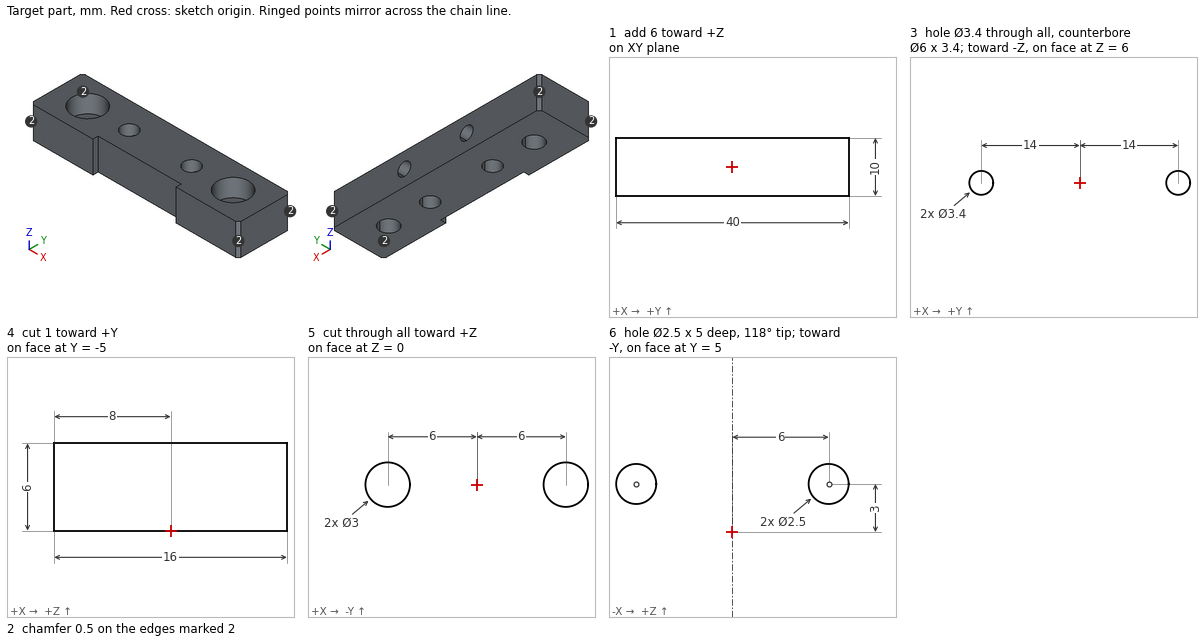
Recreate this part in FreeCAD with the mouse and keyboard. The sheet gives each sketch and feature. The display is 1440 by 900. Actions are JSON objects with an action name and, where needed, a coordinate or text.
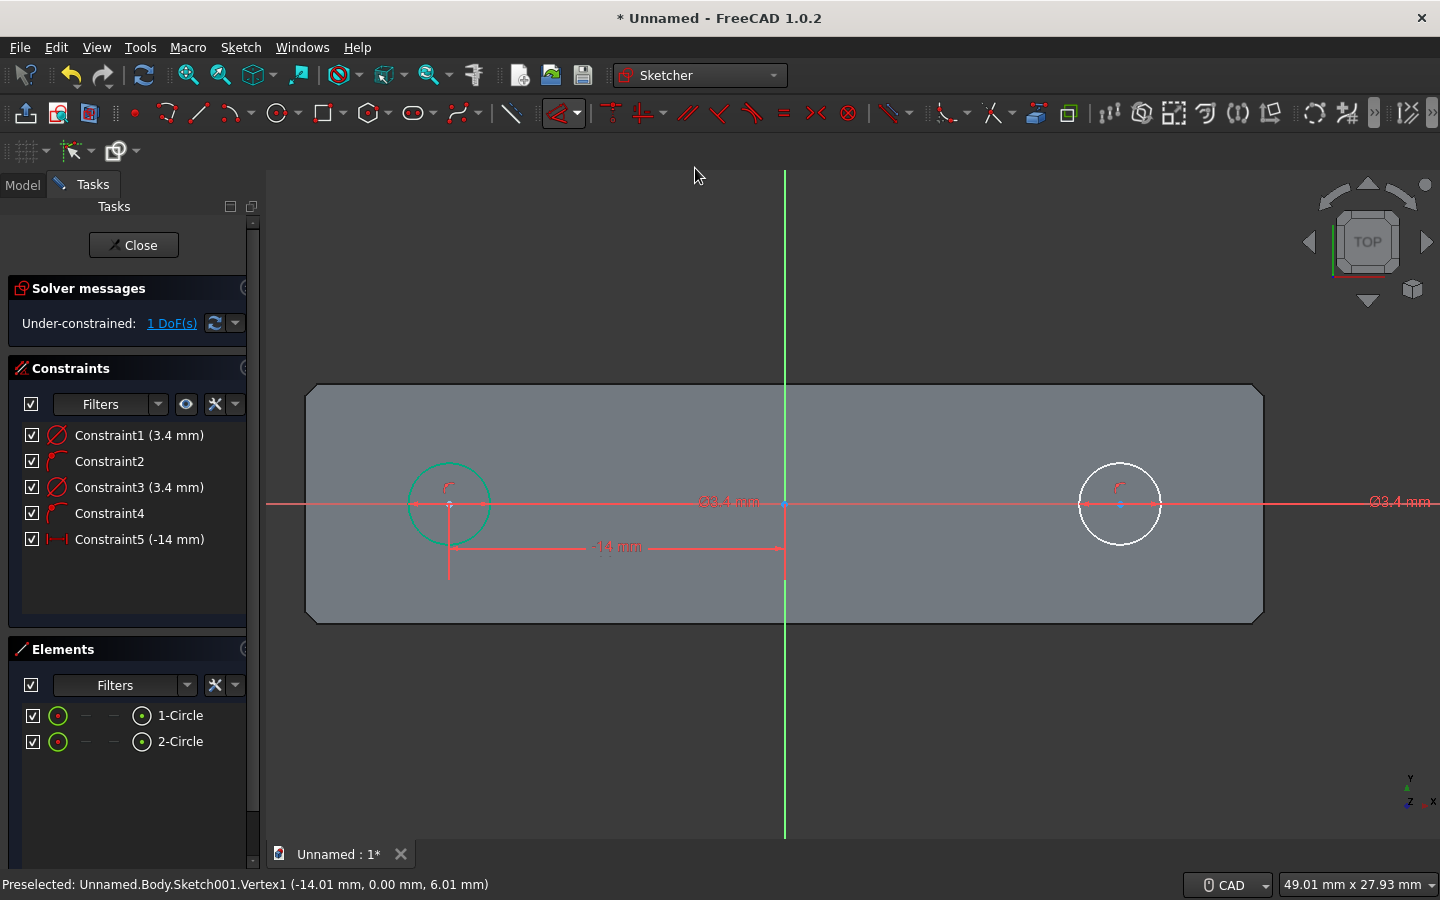
{"action": "left_click", "coordinate": [1120, 504]}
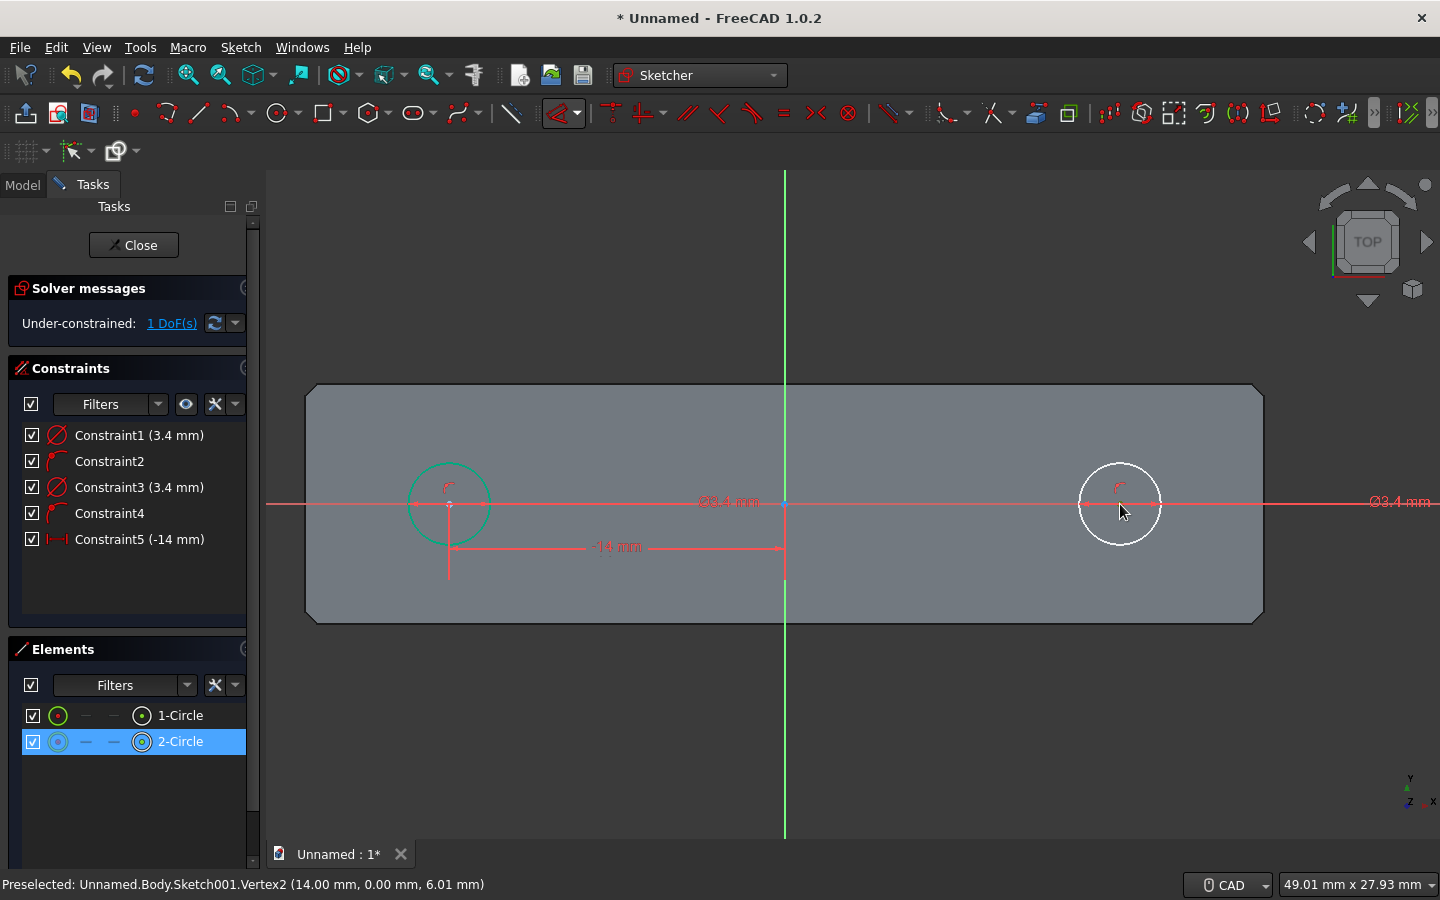
{"action": "key", "text": "l"}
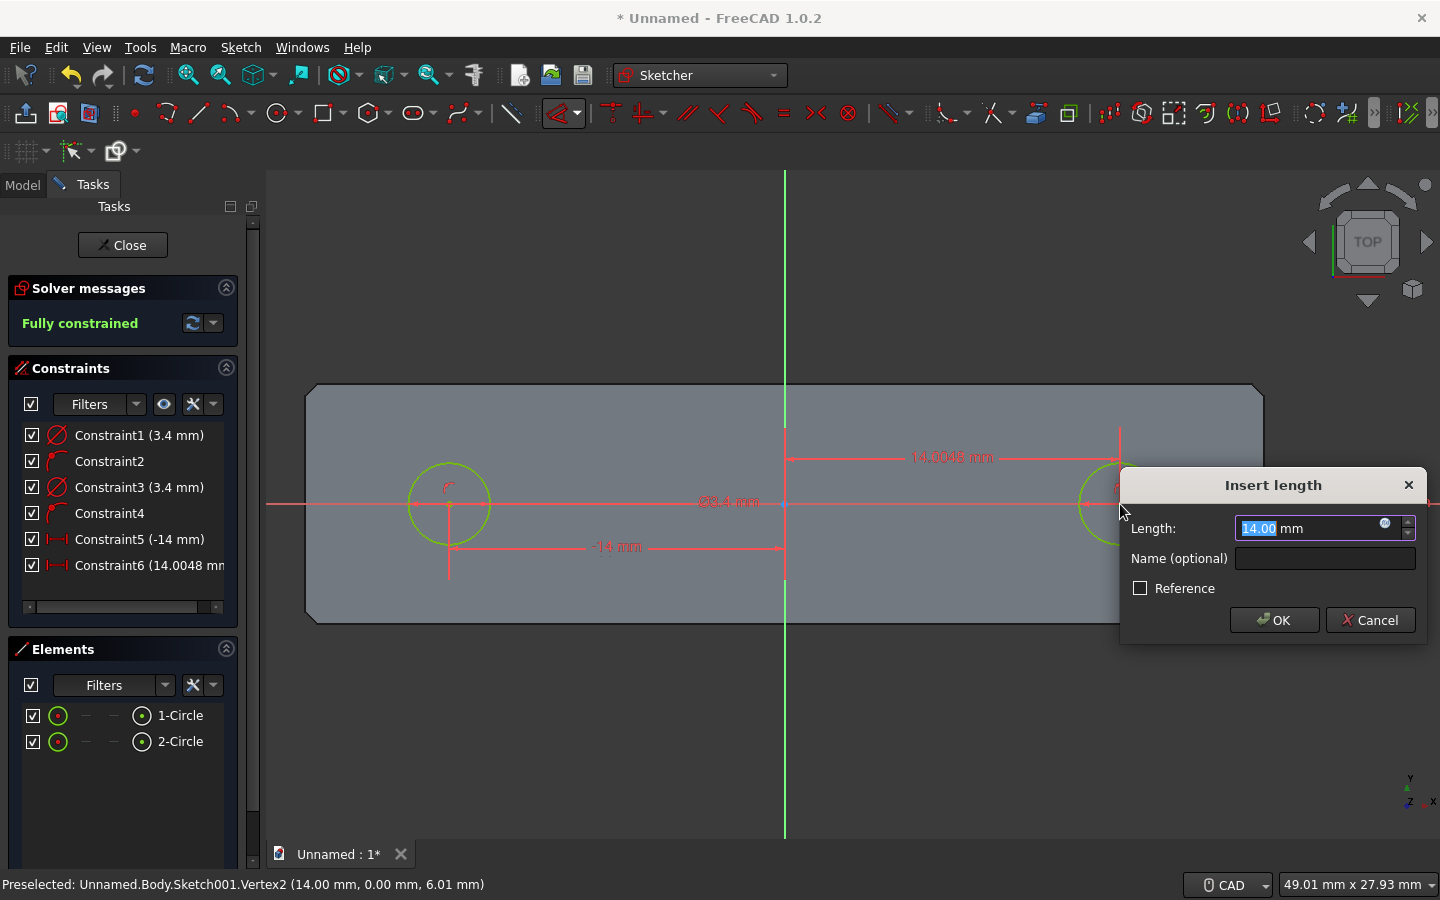
{"action": "type", "text": "14"}
{"action": "key", "text": "Return"}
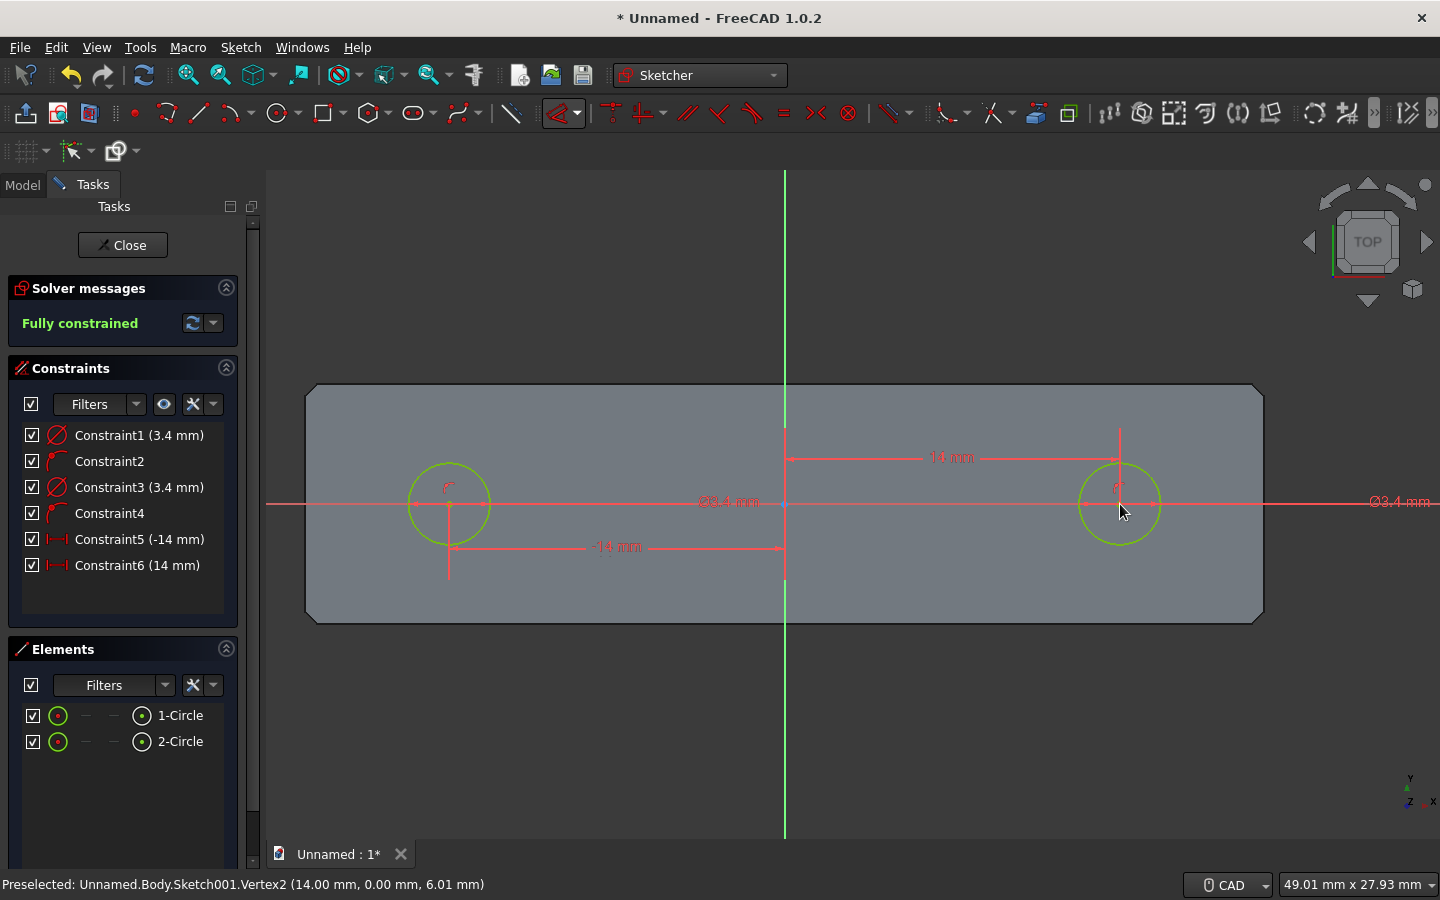
{"action": "left_click", "coordinate": [123, 245]}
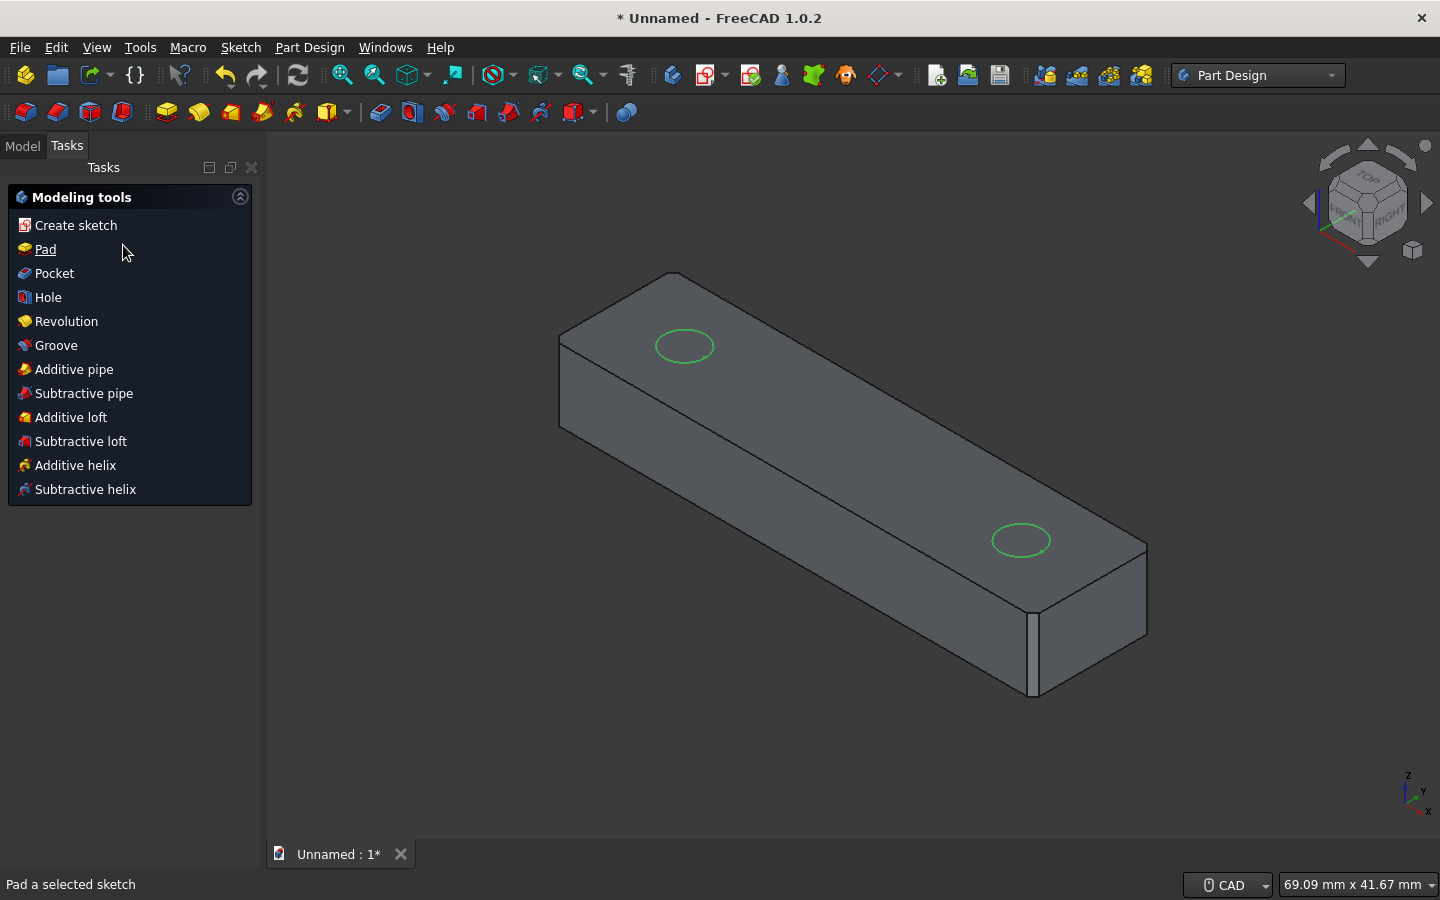
{"action": "left_click", "coordinate": [414, 112]}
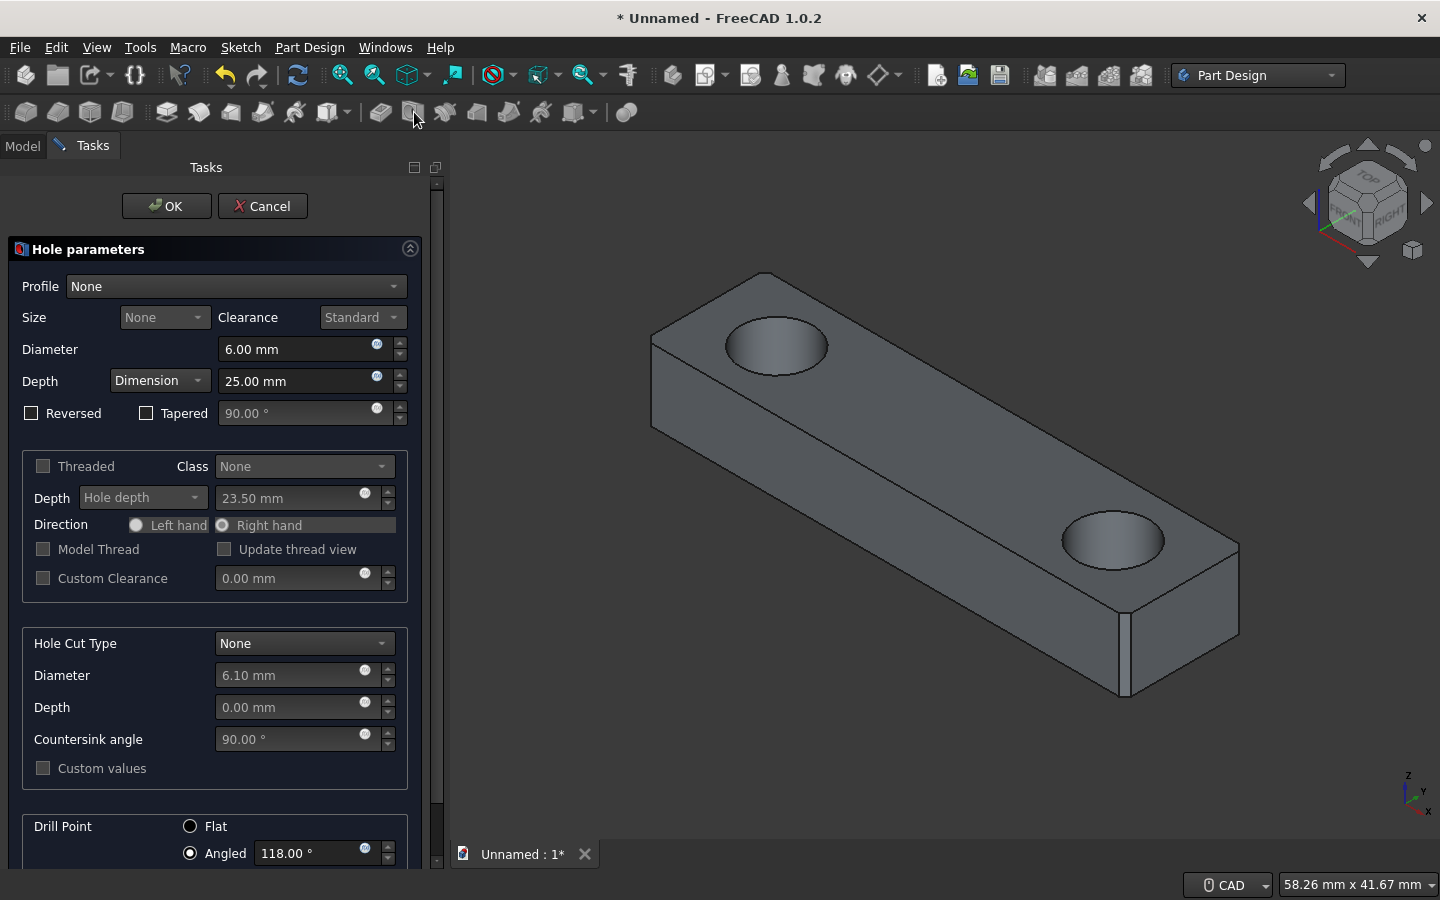
{"action": "triple_click", "coordinate": [305, 349]}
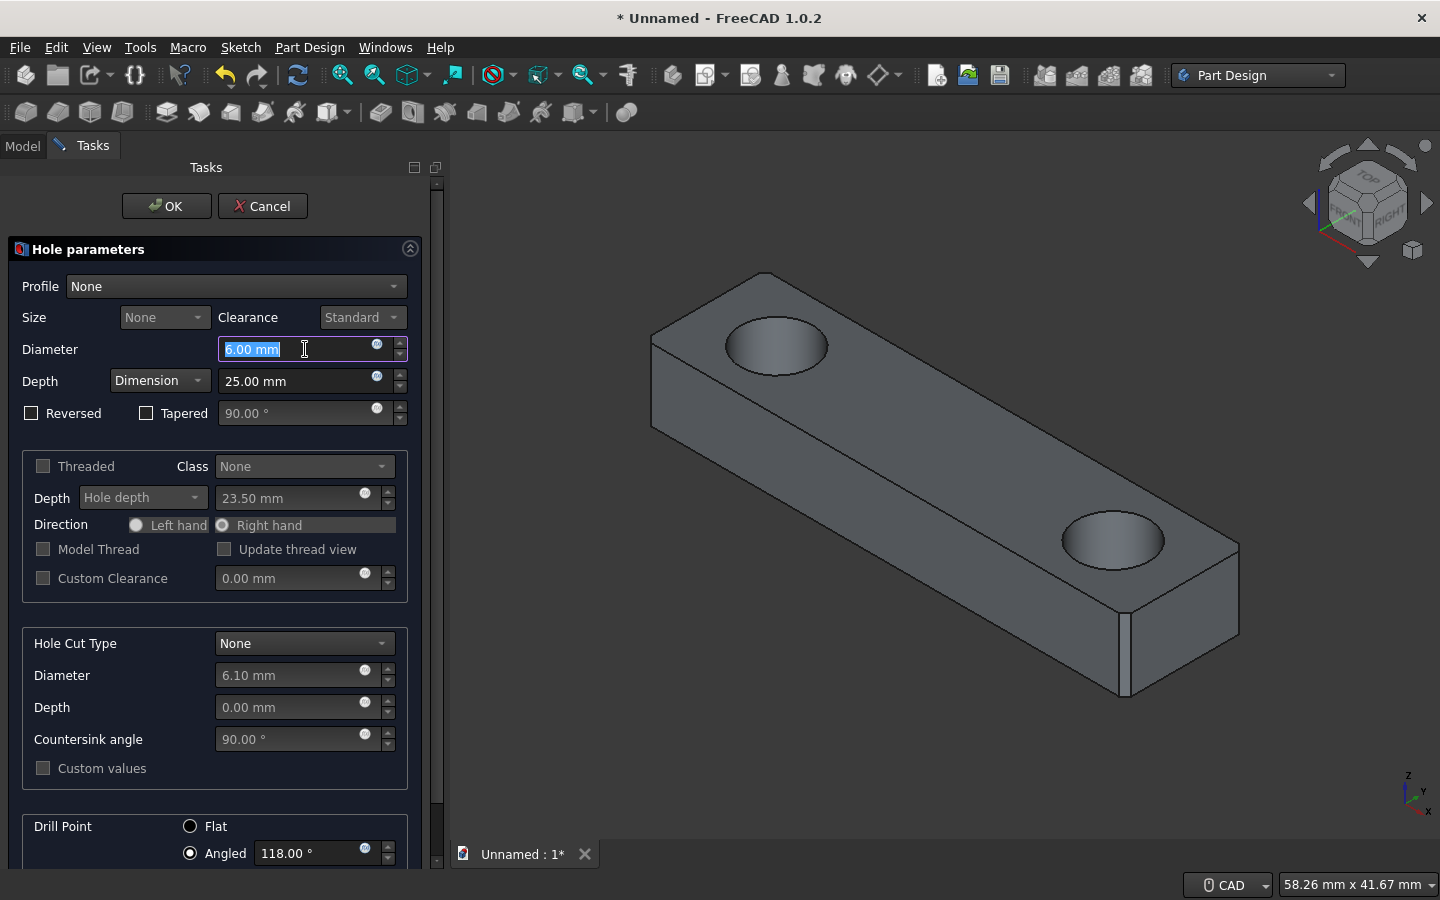
{"action": "type", "text": "3.4"}
{"action": "key", "text": "Tab"}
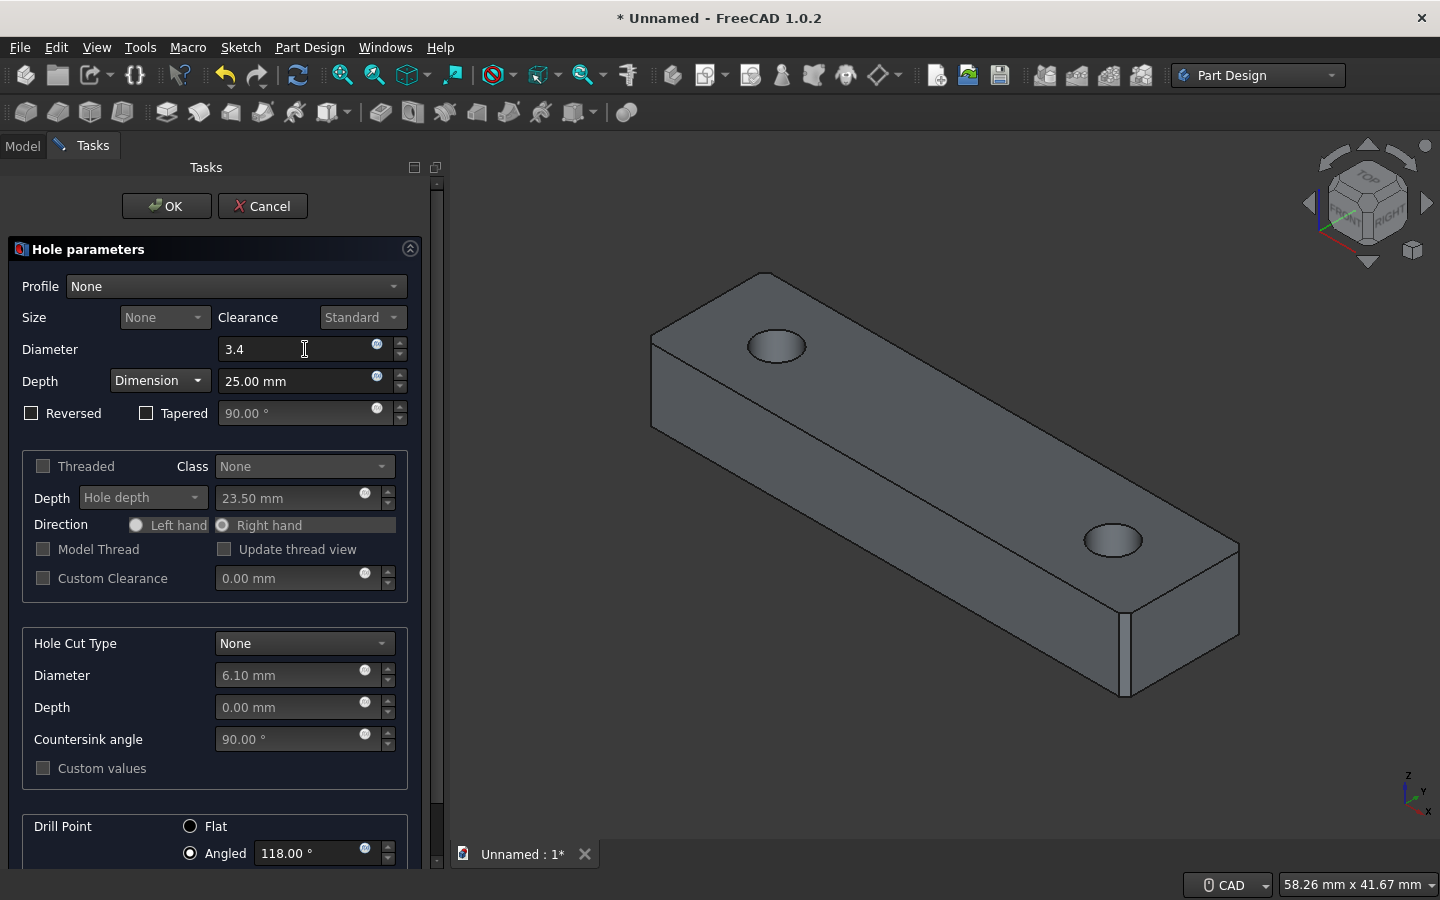
{"action": "left_click", "coordinate": [161, 380]}